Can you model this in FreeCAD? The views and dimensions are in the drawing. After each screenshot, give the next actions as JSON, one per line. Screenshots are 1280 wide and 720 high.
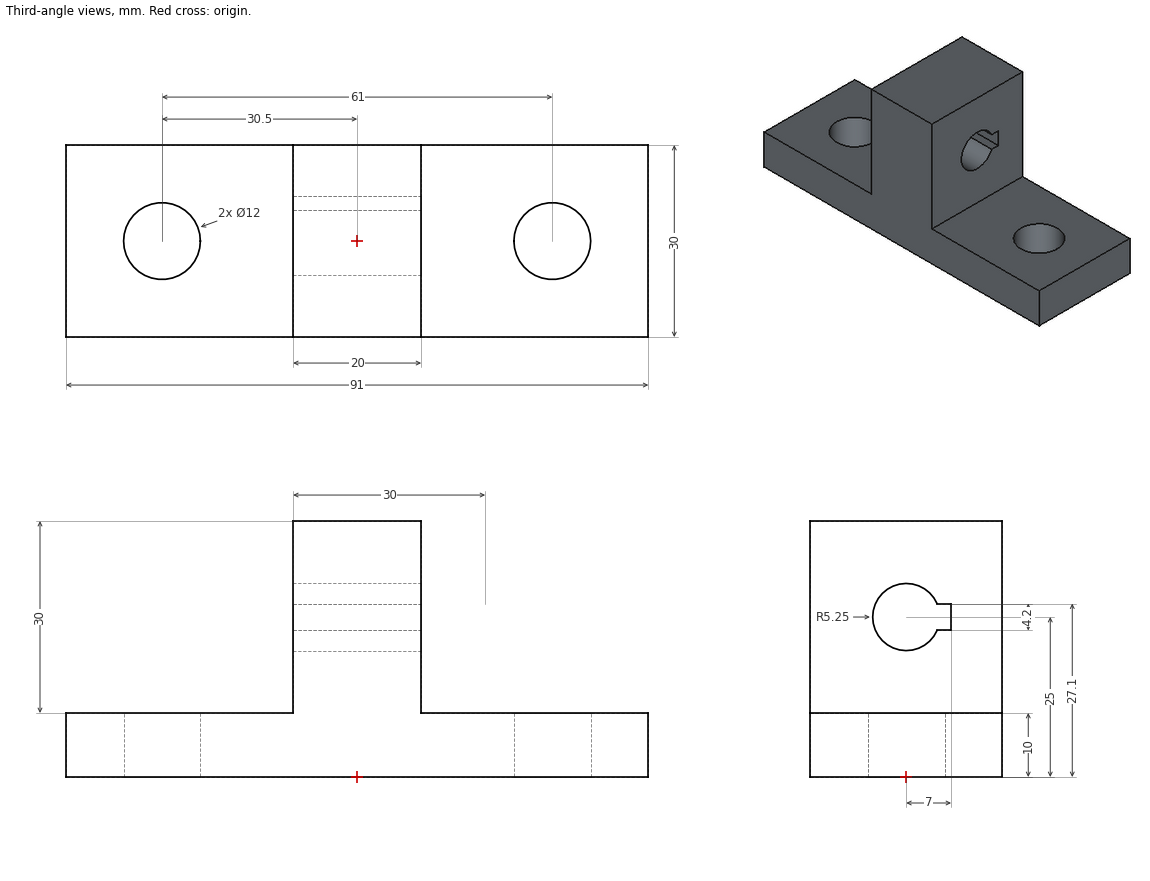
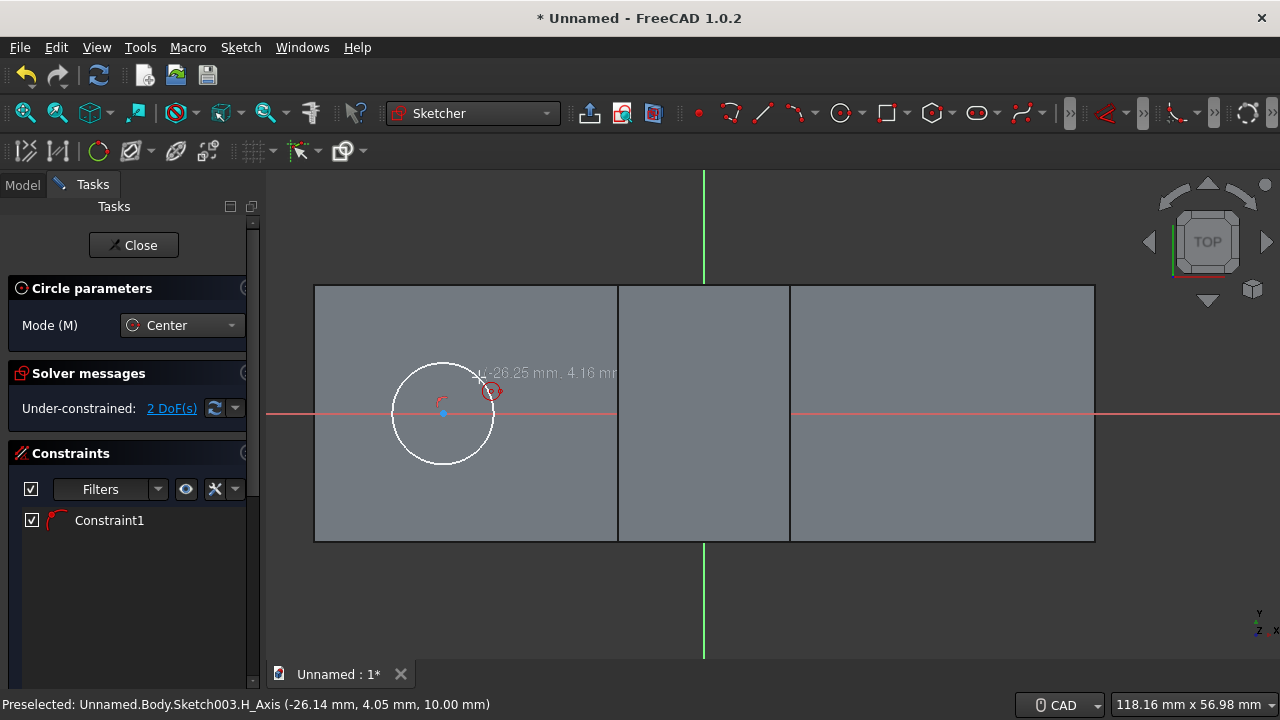
{"action": "left_click", "coordinate": [966, 414]}
{"action": "left_click", "coordinate": [1002, 377]}
{"action": "key", "text": "Escape"}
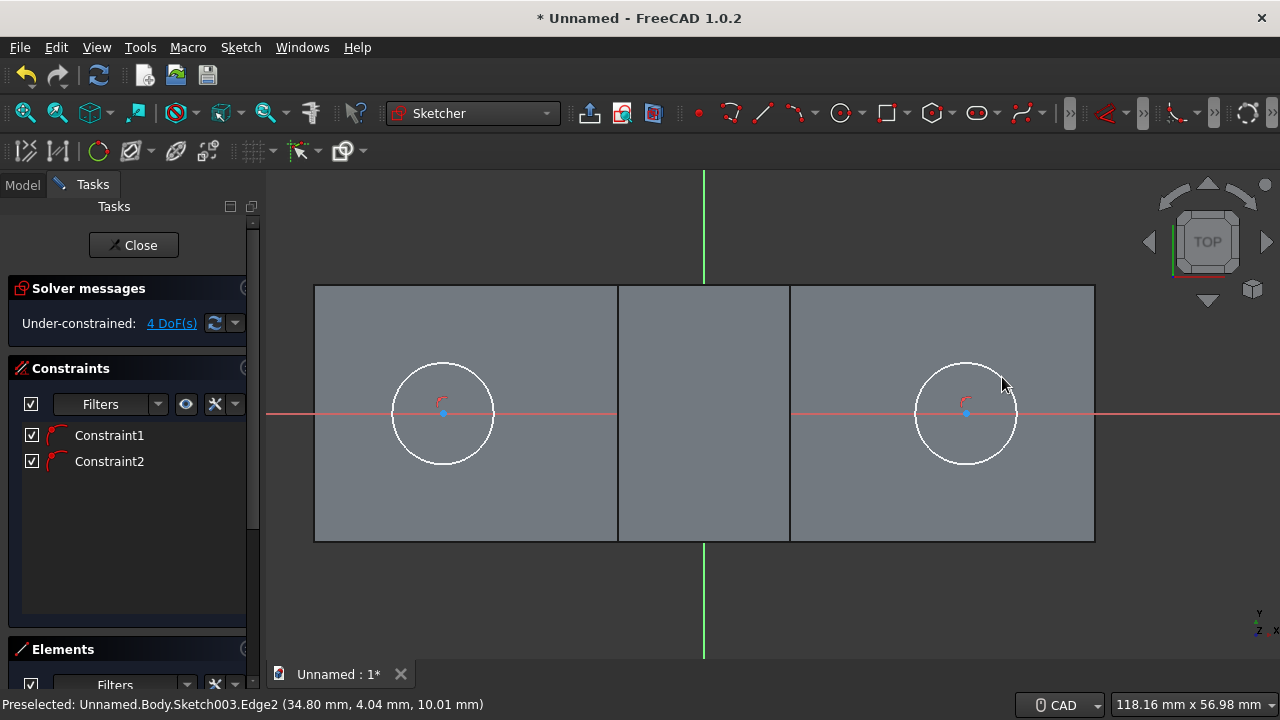
{"action": "left_click", "coordinate": [479, 378]}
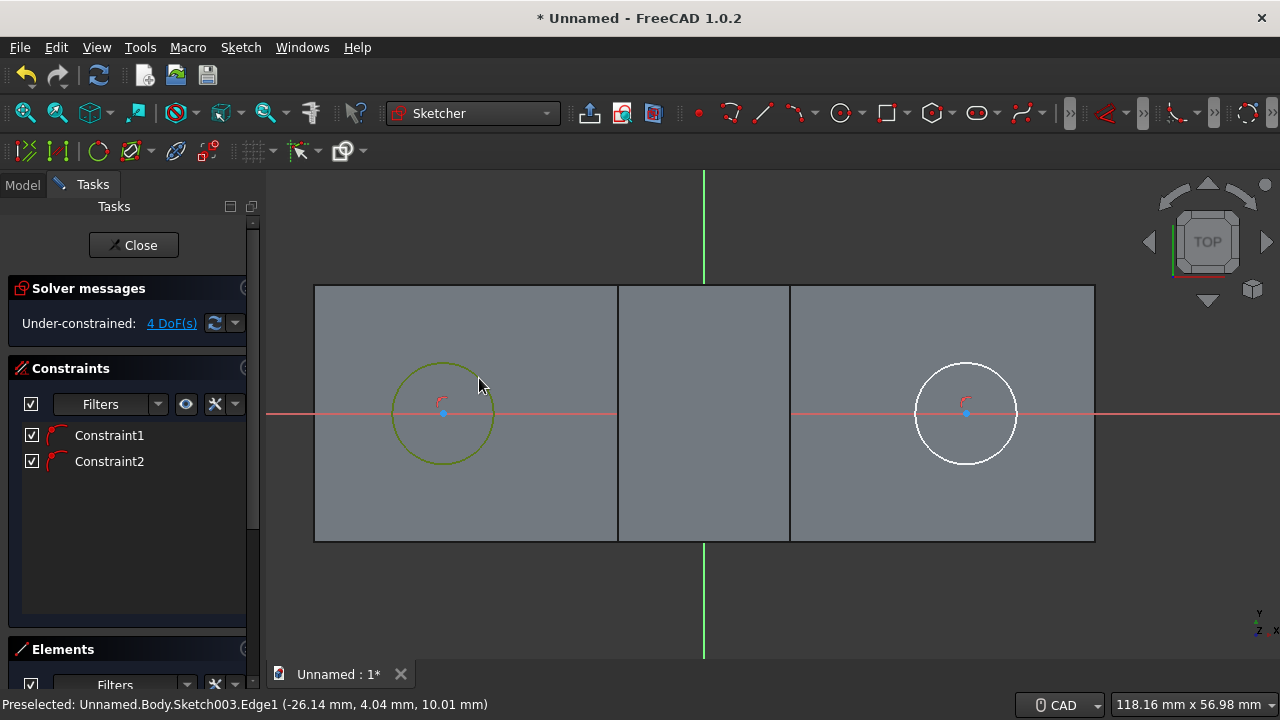
{"action": "left_click", "coordinate": [1002, 378]}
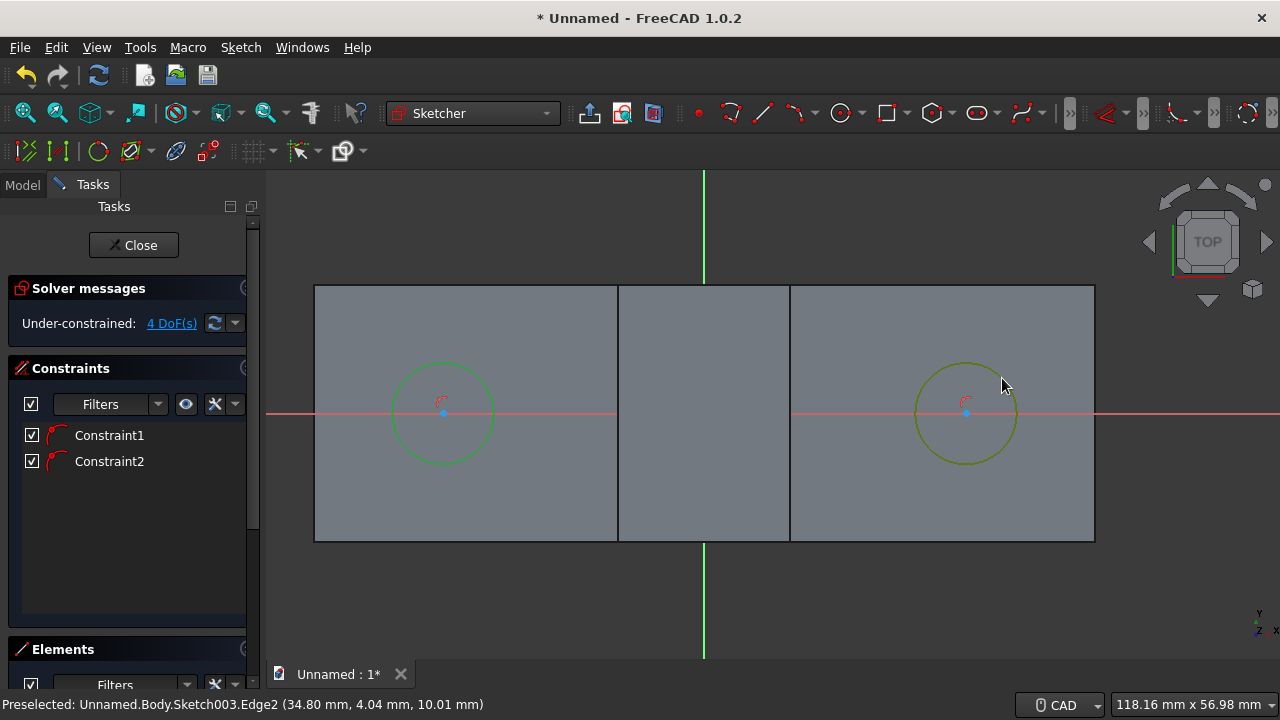
{"action": "key", "text": "e"}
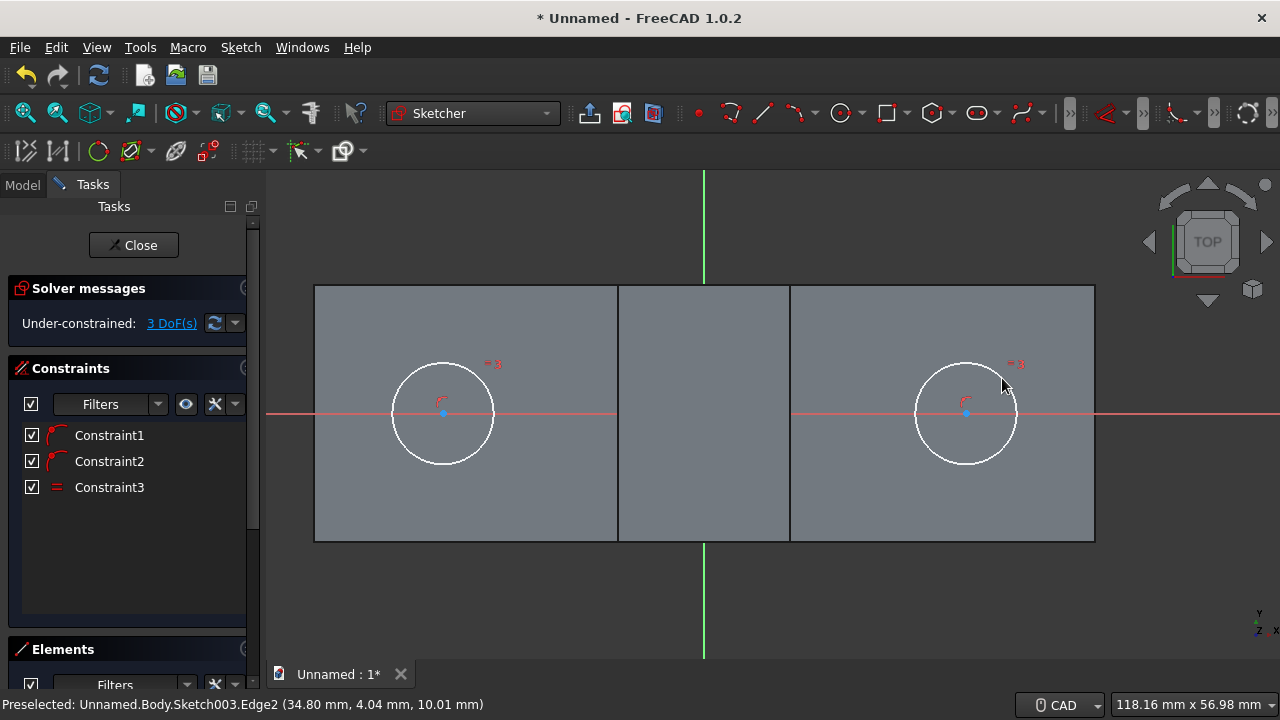
{"action": "key", "text": "d"}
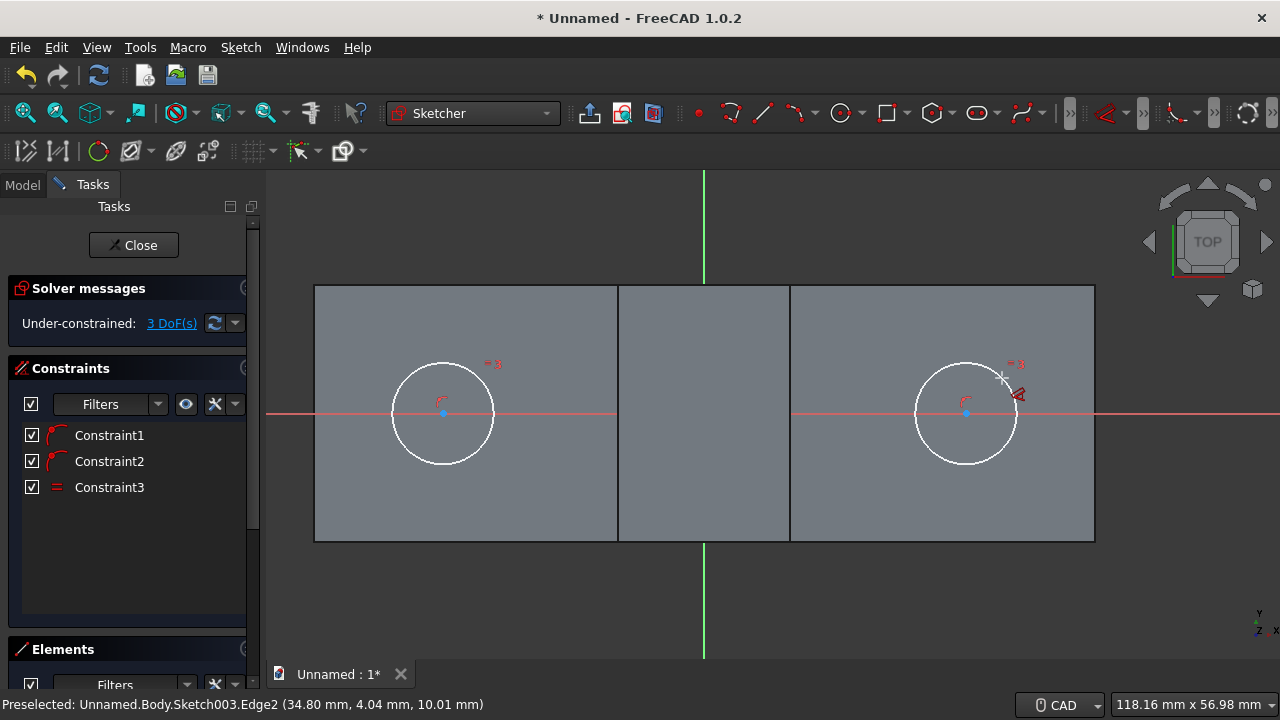
{"action": "left_click", "coordinate": [479, 378]}
{"action": "left_click", "coordinate": [502, 355]}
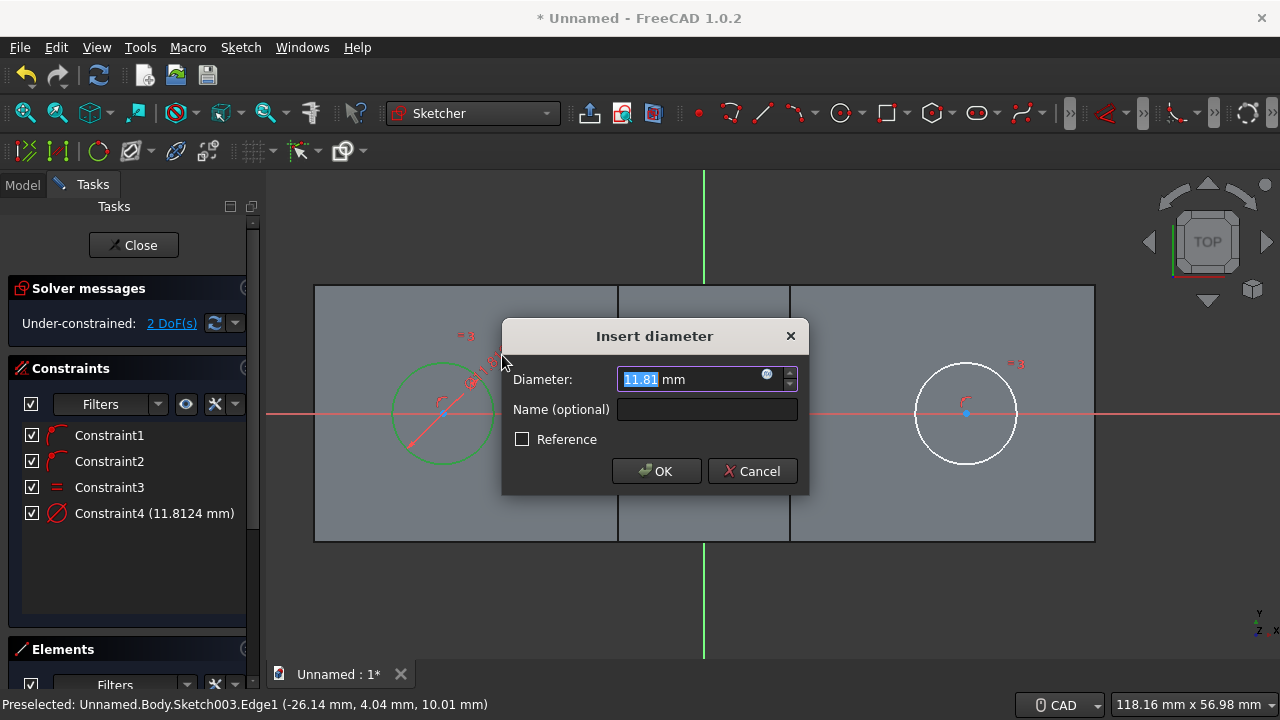
{"action": "type", "text": "12"}
{"action": "key", "text": "Return"}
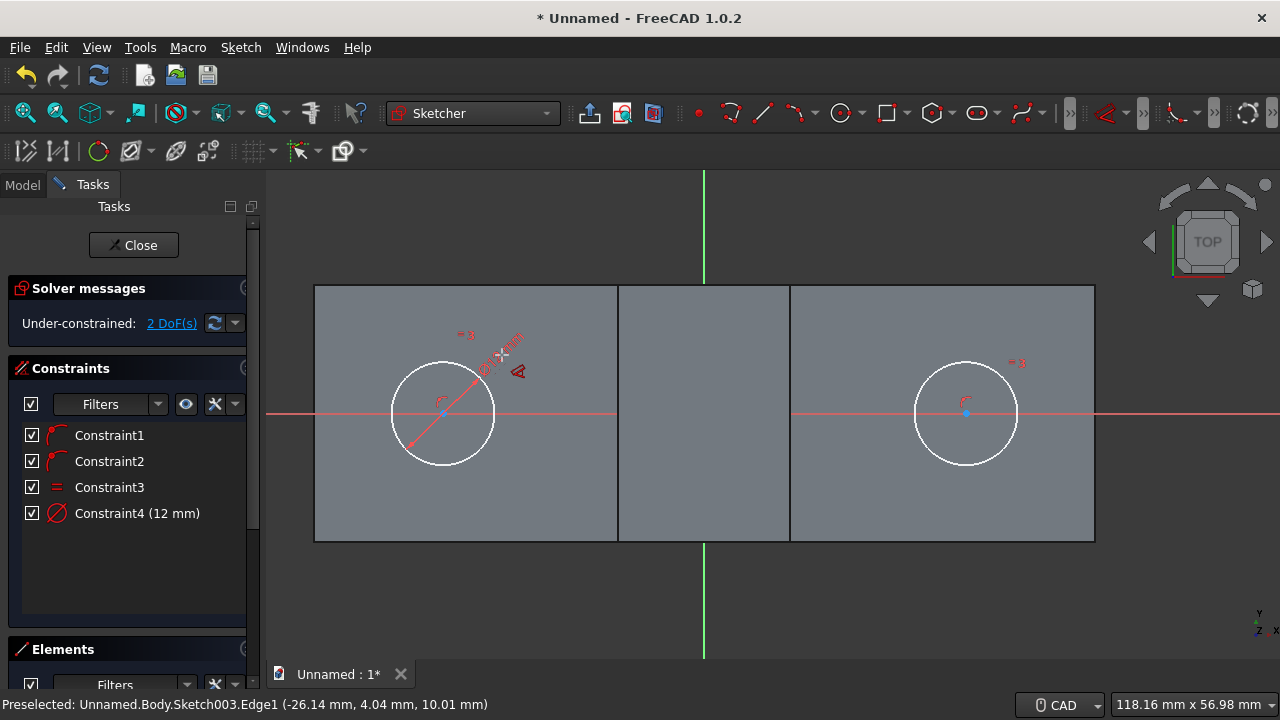
{"action": "left_click", "coordinate": [443, 414]}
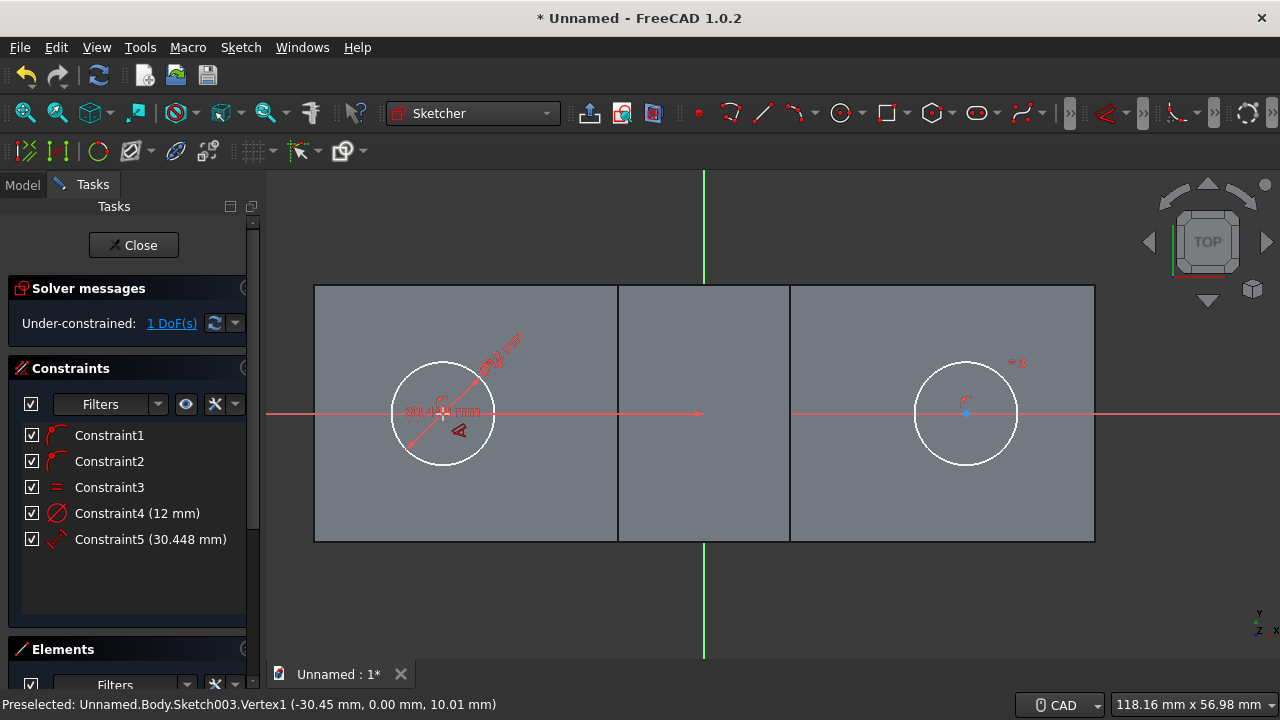
{"action": "left_click", "coordinate": [966, 414]}
{"action": "left_click", "coordinate": [584, 448]}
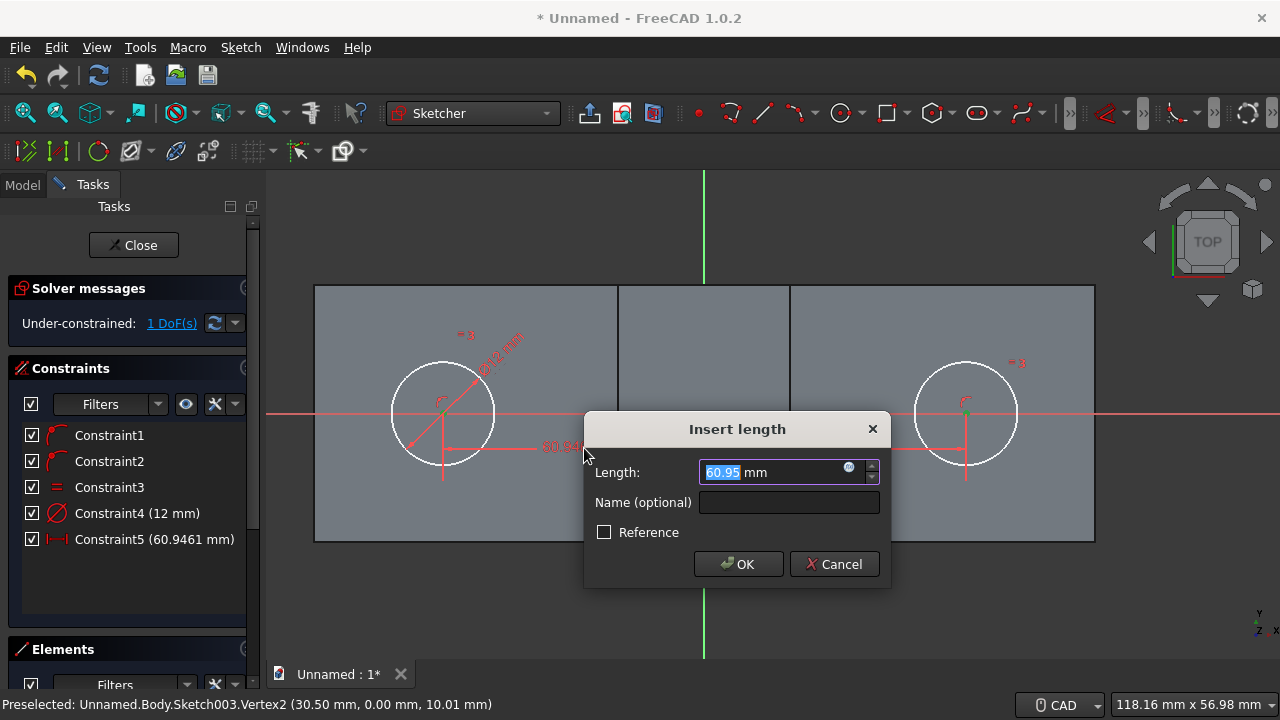
{"action": "type", "text": "61"}
{"action": "key", "text": "Return"}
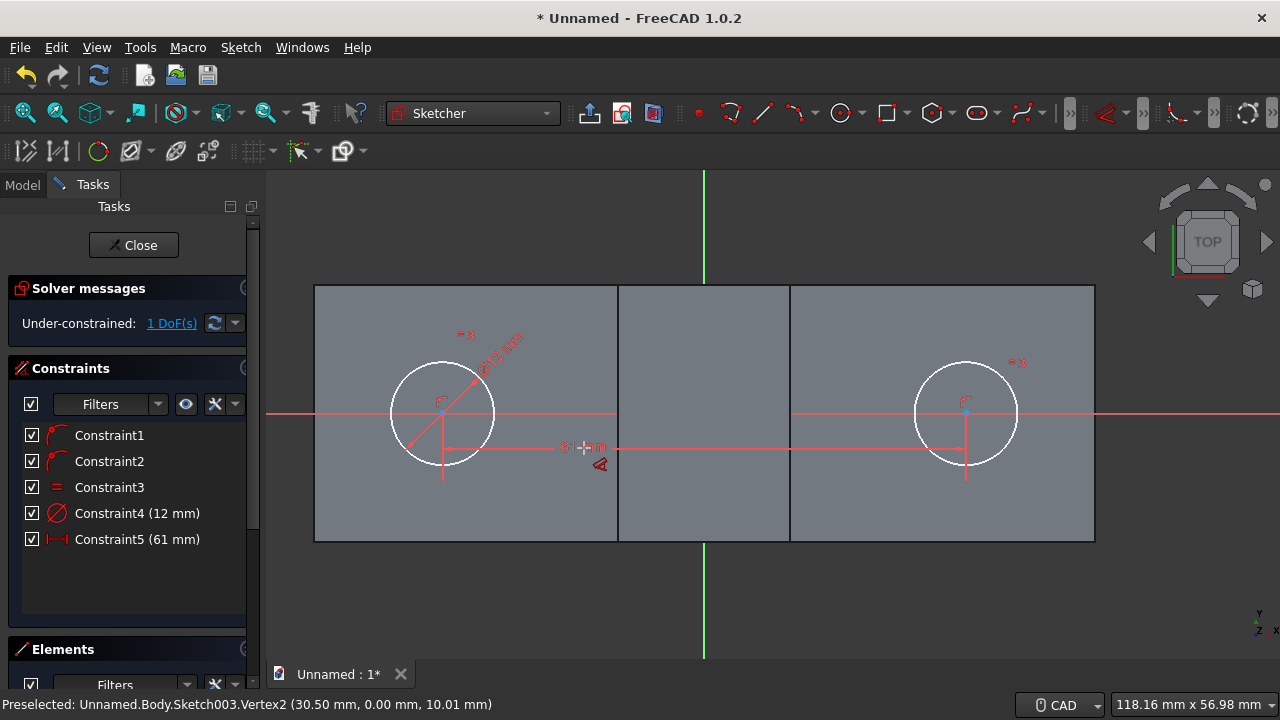
{"action": "left_click", "coordinate": [443, 414]}
{"action": "left_click", "coordinate": [513, 448]}